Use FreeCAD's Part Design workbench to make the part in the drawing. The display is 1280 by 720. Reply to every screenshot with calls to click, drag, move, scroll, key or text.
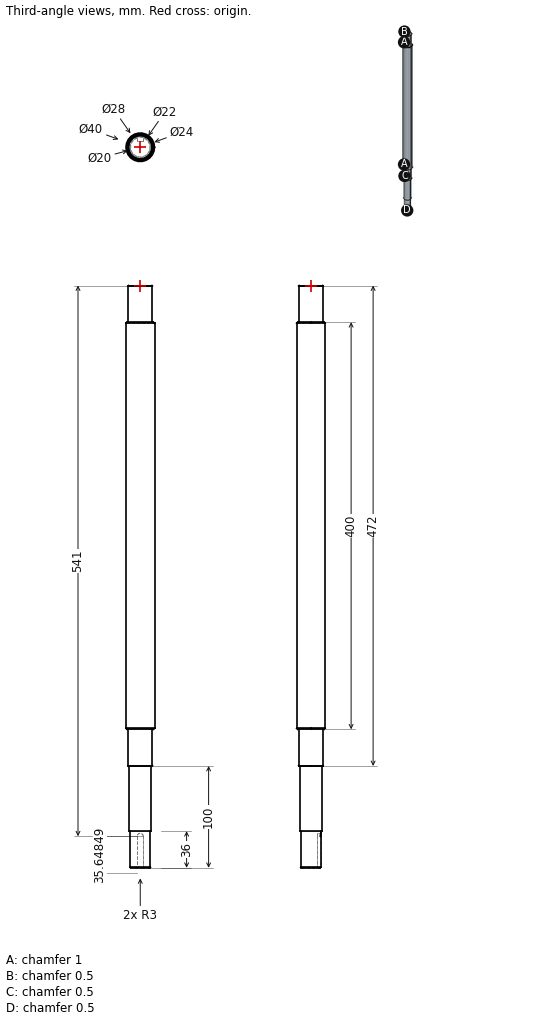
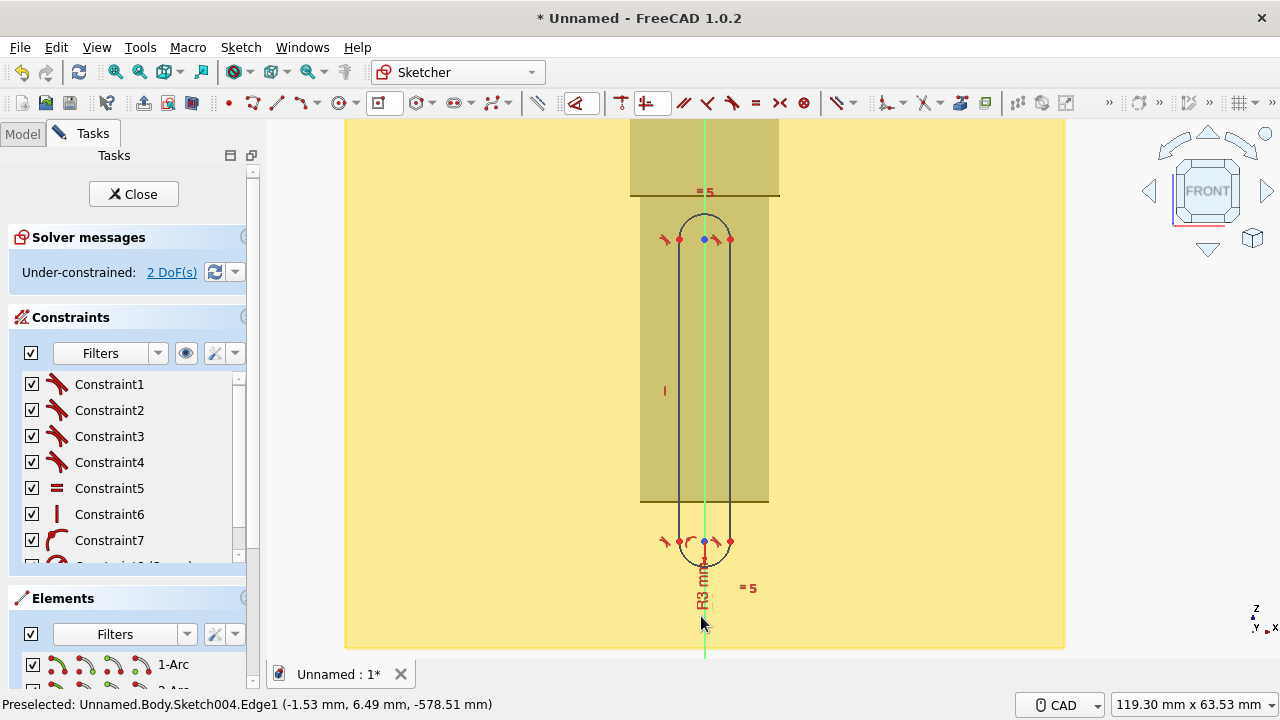
click(730, 240)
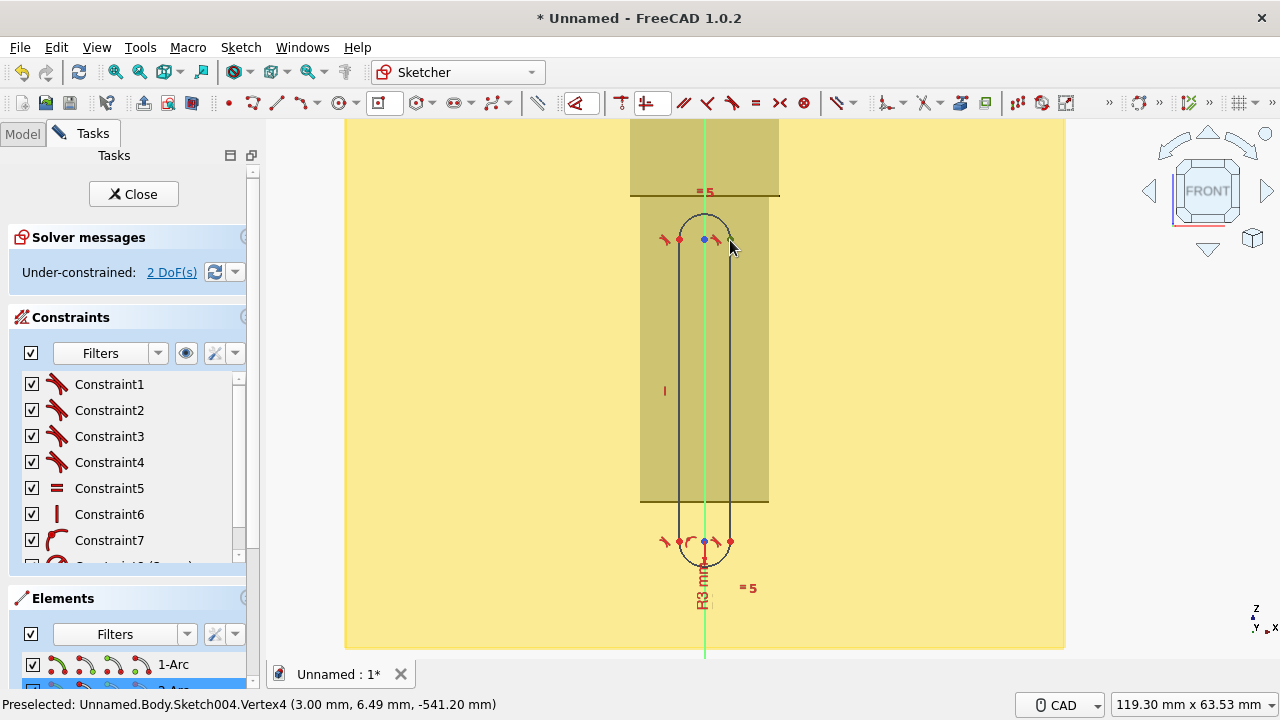
click(594, 104)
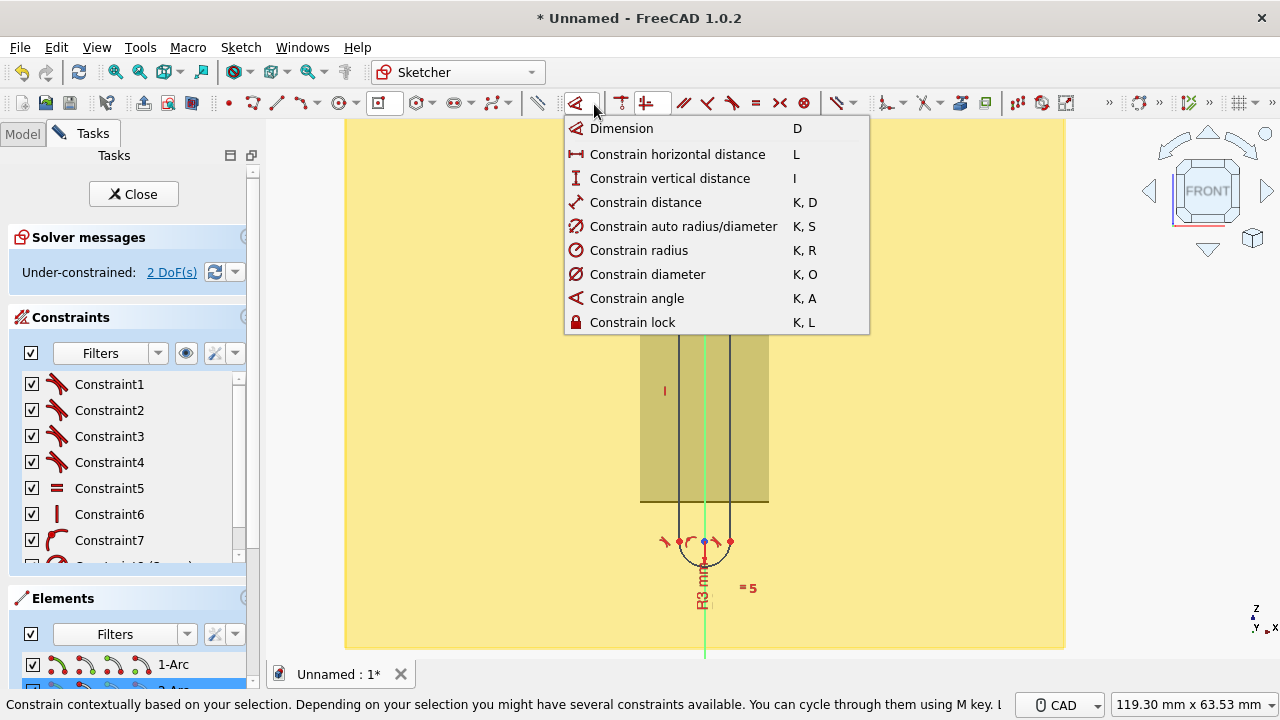
click(717, 178)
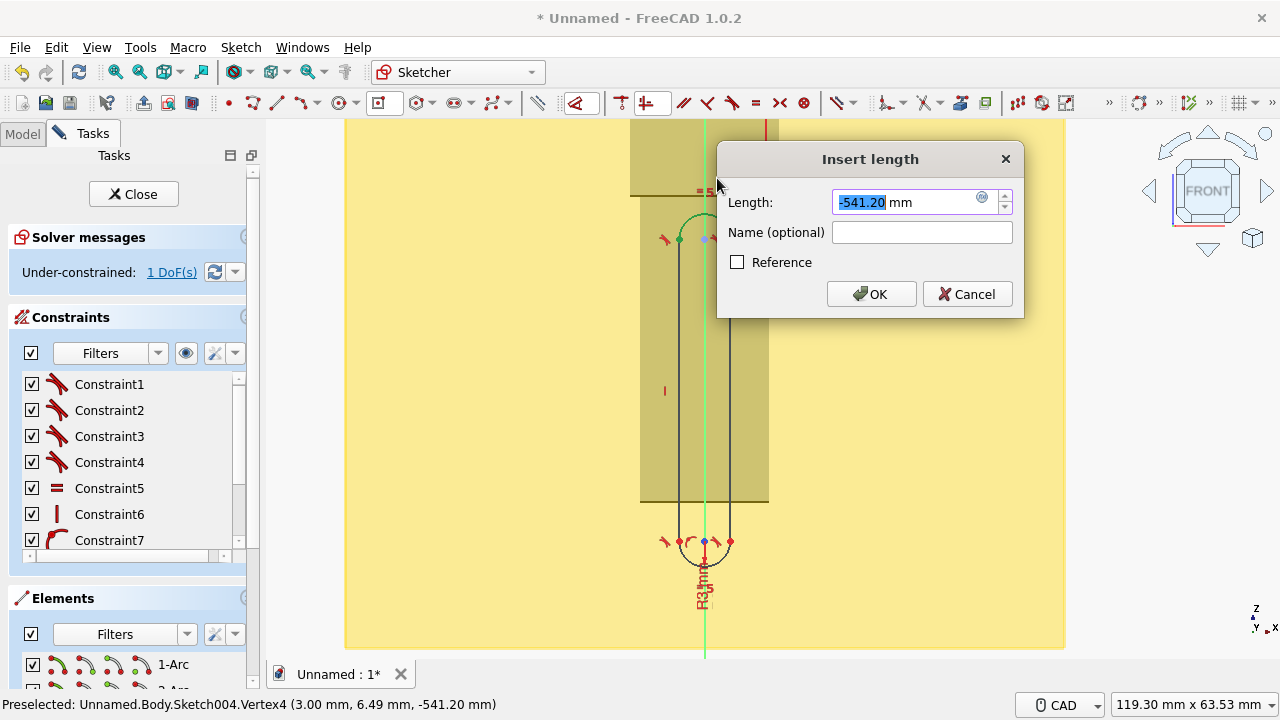
text(-541)
key(Return)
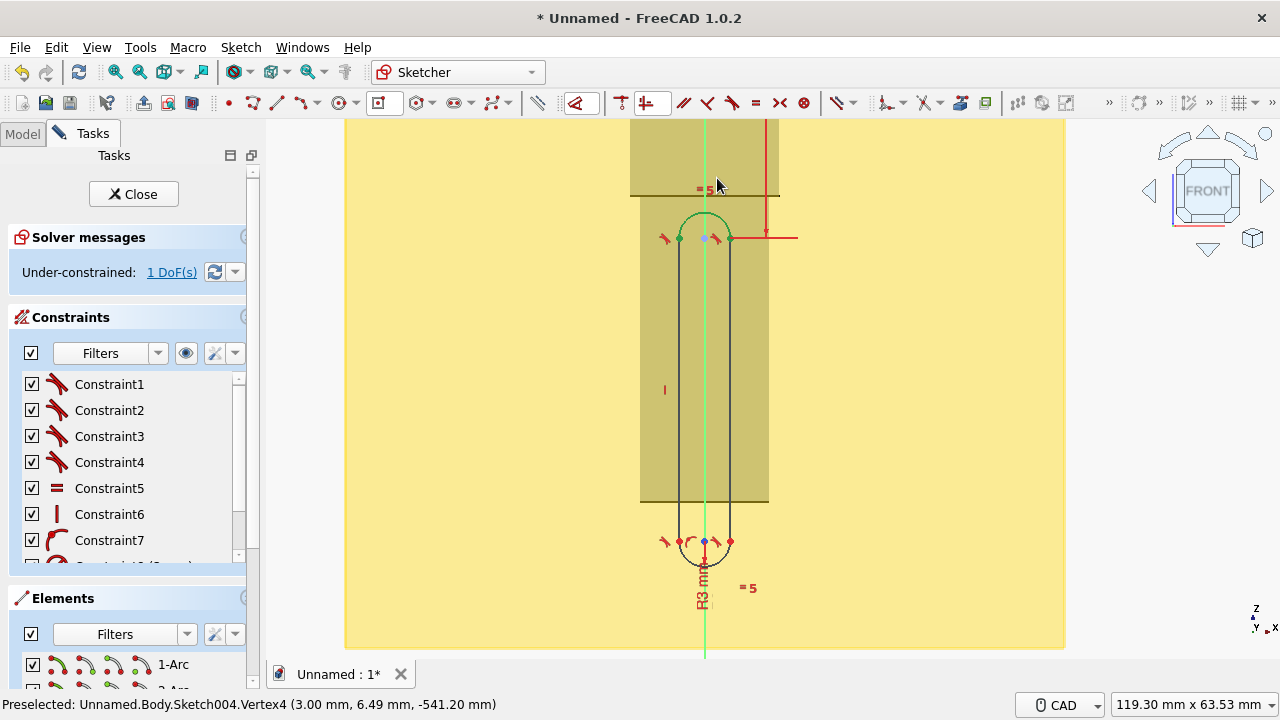
click(679, 450)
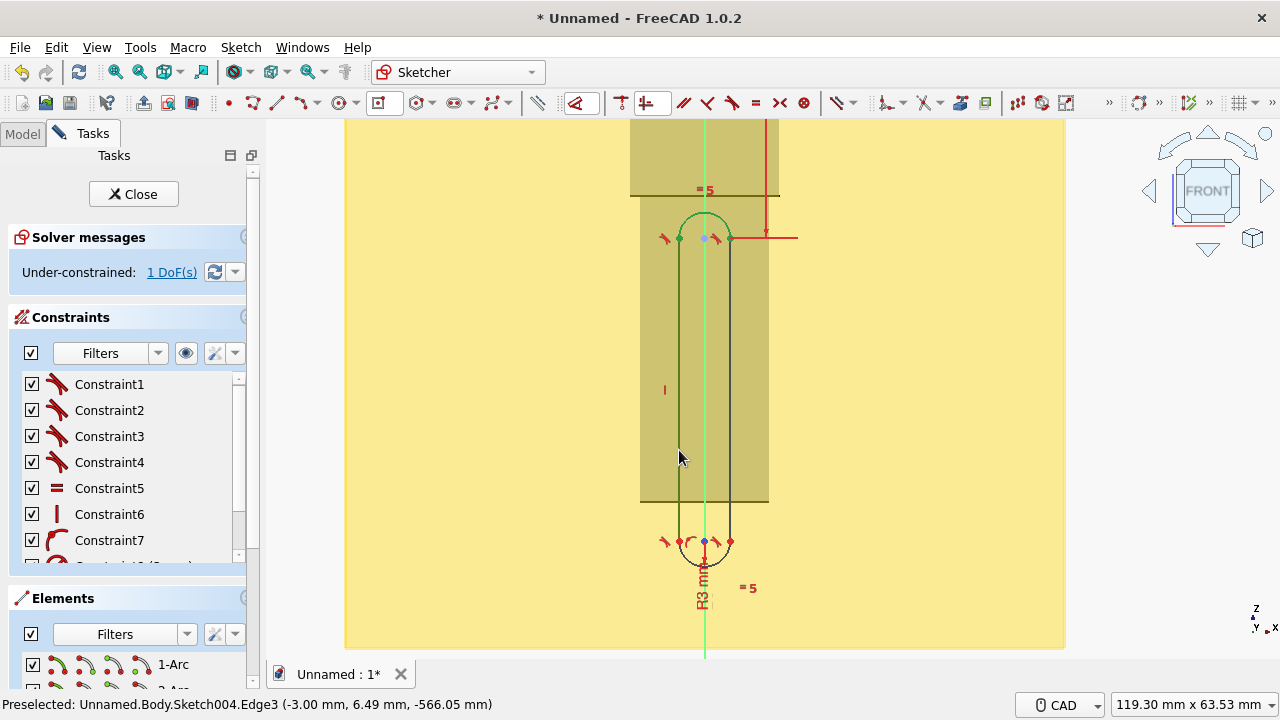
key(i)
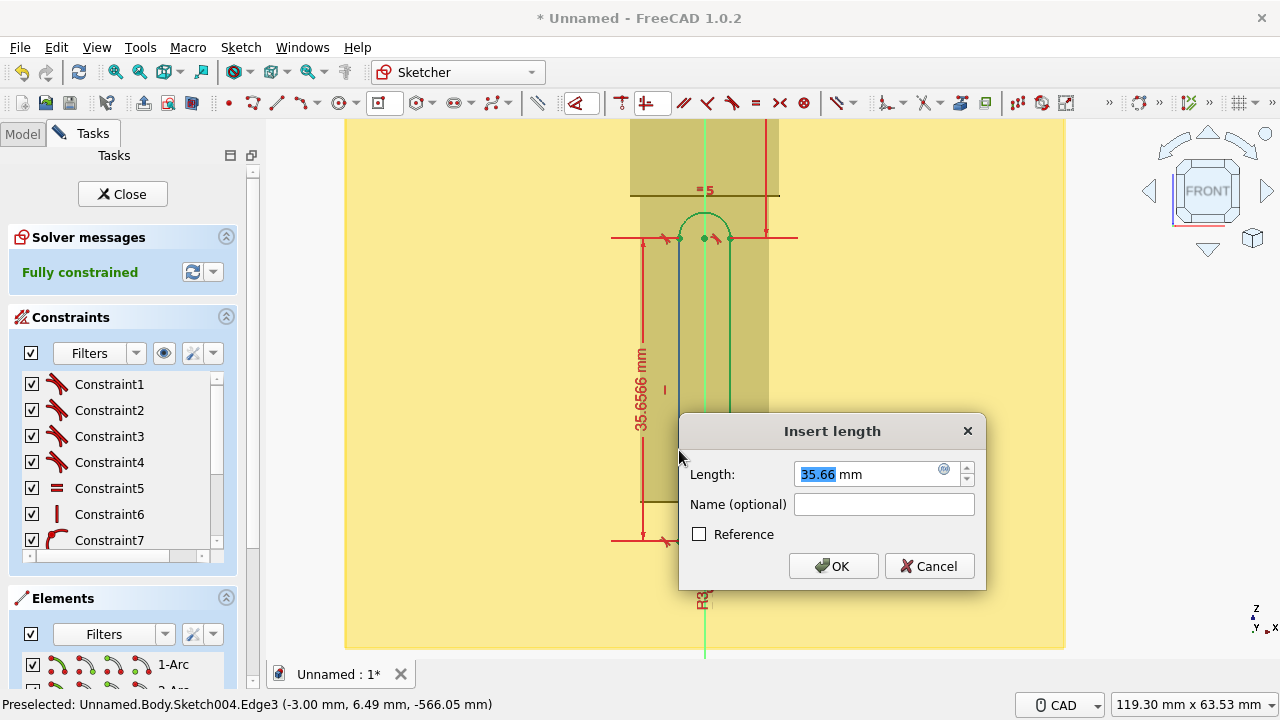
text(35.64849)
key(Return)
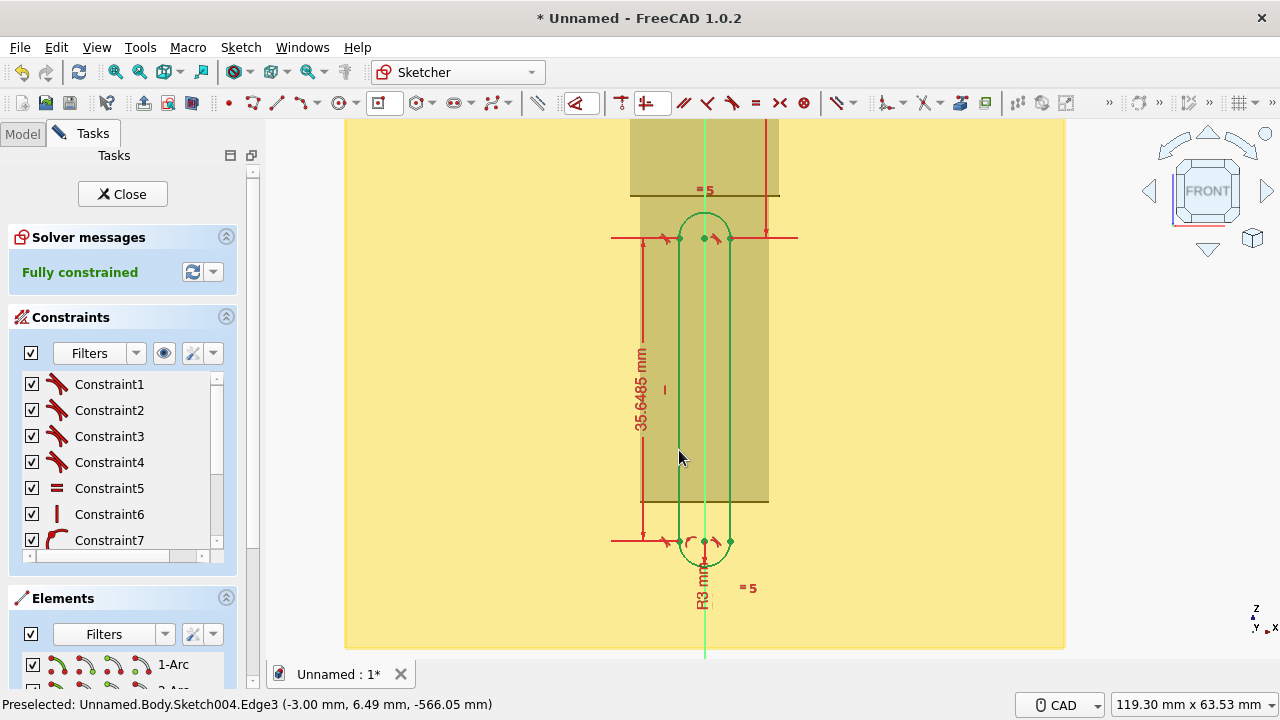
click(123, 194)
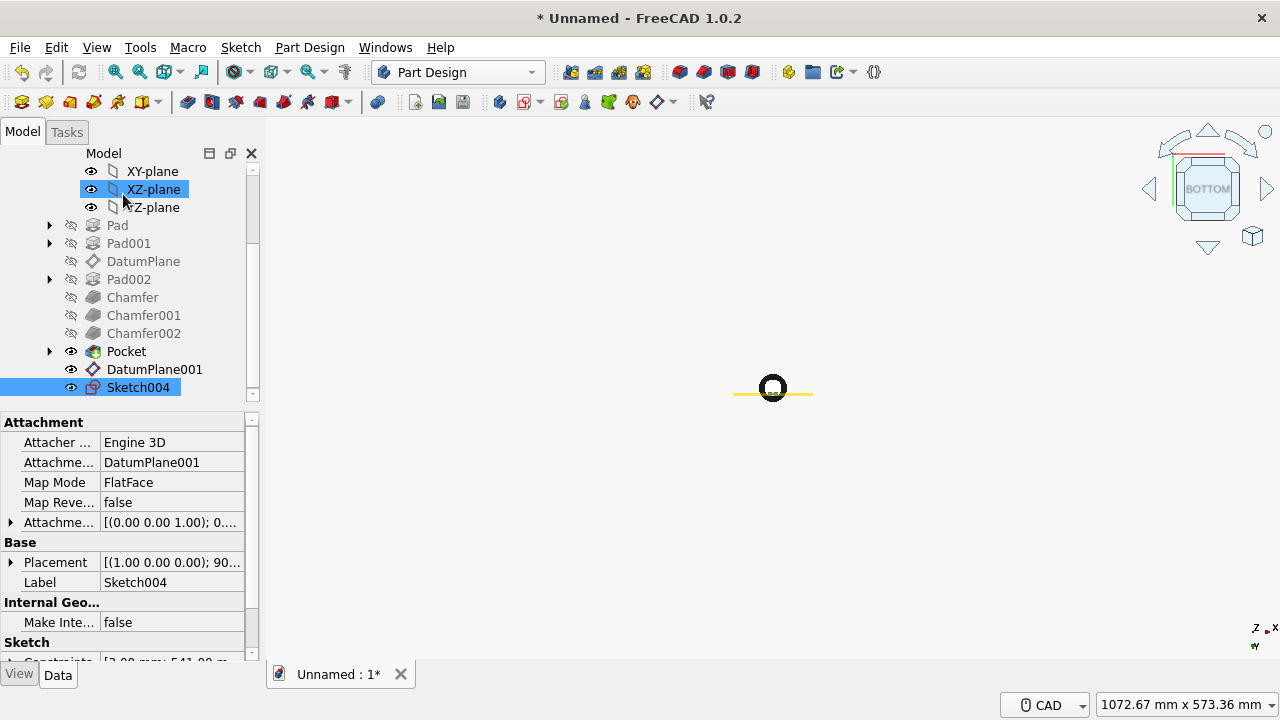
click(188, 102)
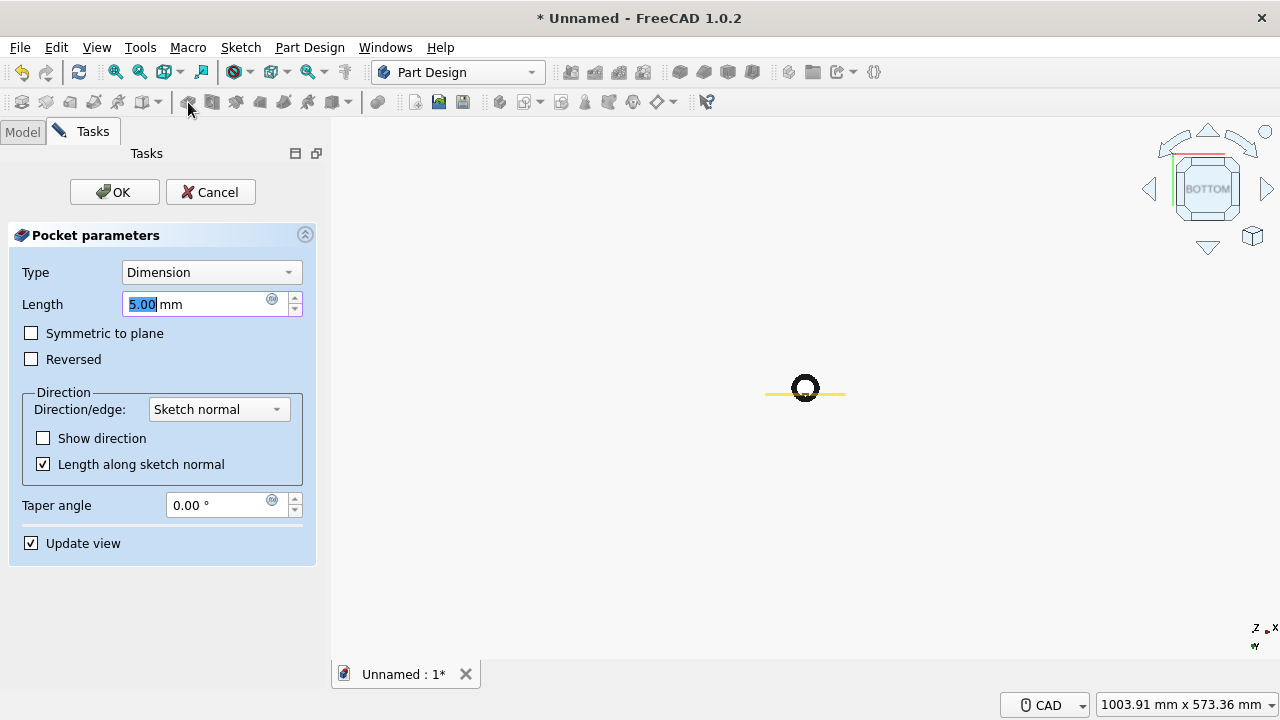
click(212, 272)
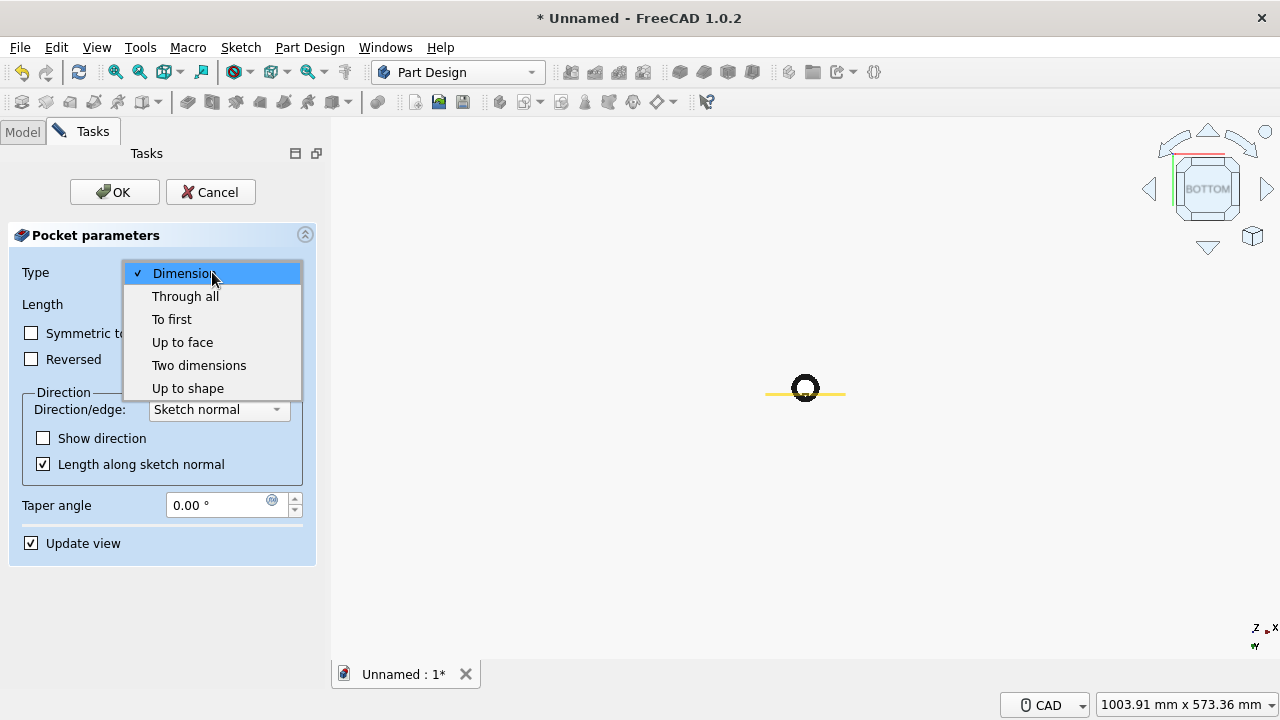
click(212, 296)